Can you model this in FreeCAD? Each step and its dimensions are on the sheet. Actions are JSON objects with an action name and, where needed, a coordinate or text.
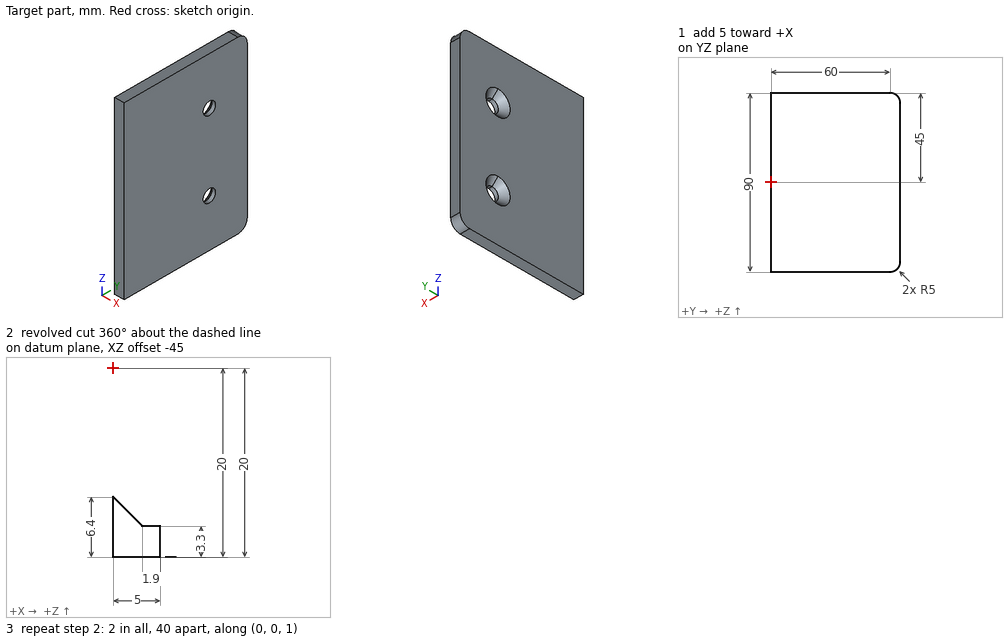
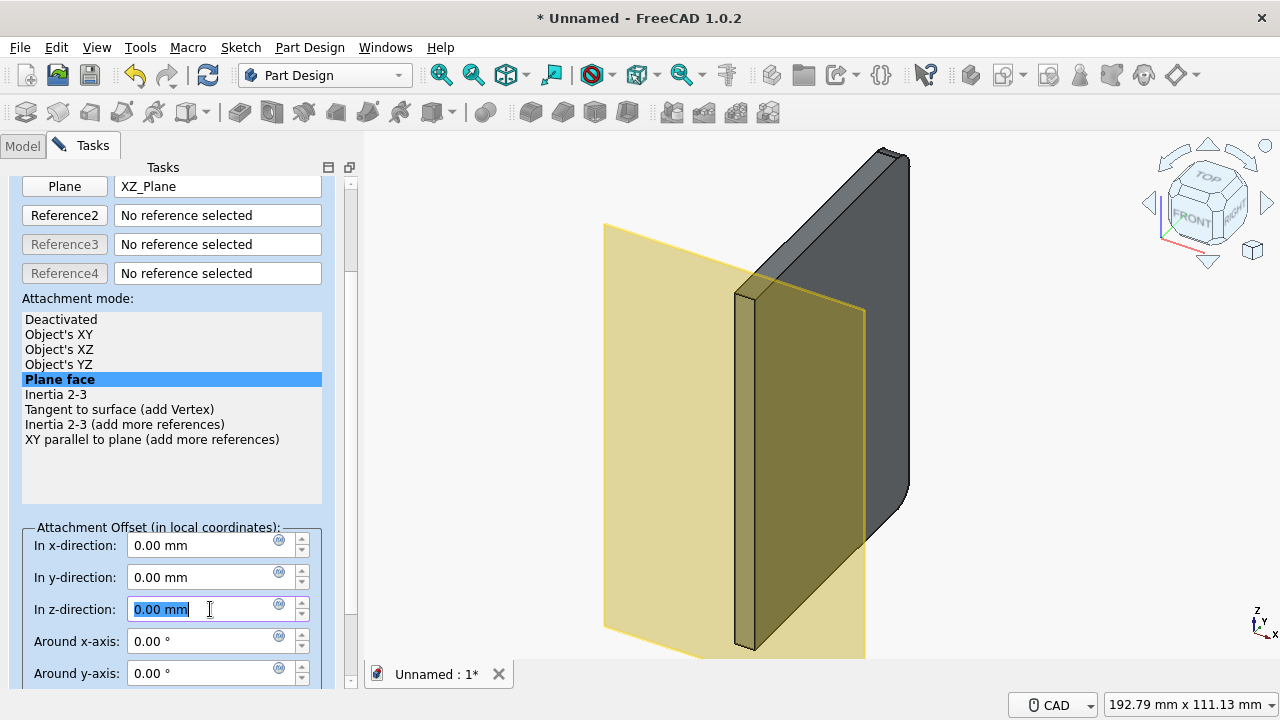
{"action": "type", "text": "-45"}
{"action": "key", "text": "Tab"}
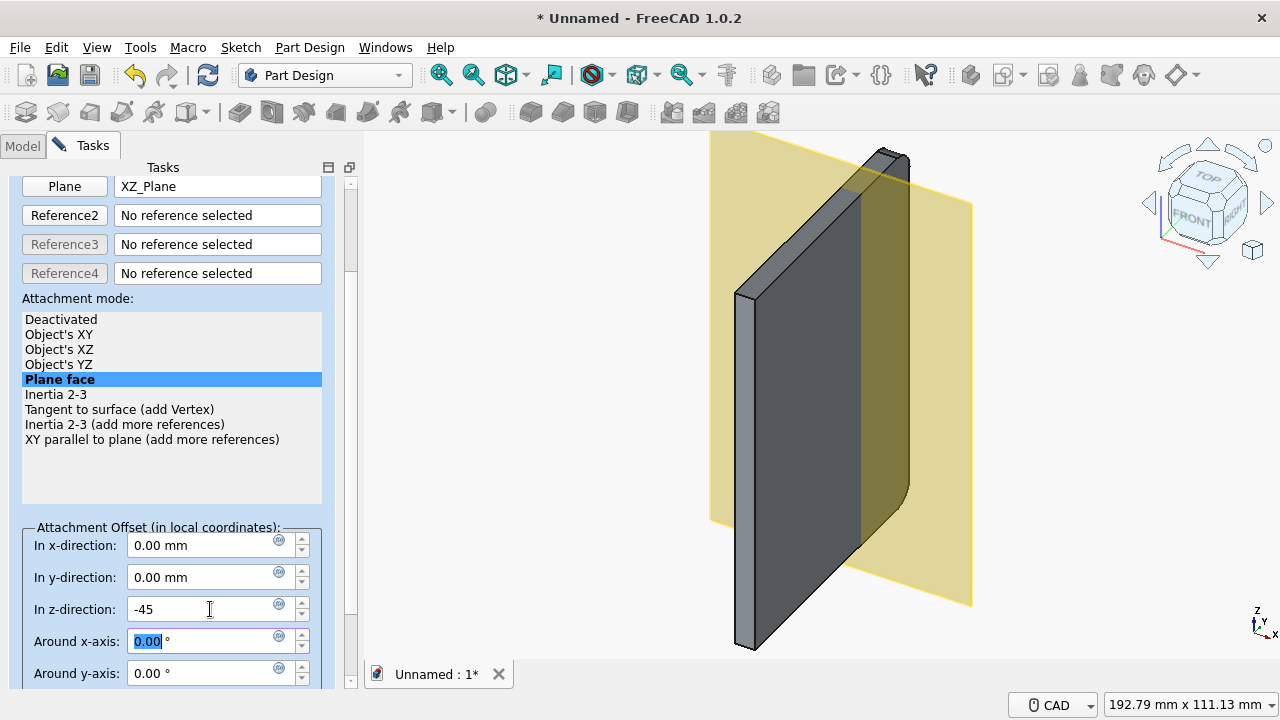
{"action": "scroll", "coordinate": [351, 432], "scroll_direction": "up", "scroll_amount": 3}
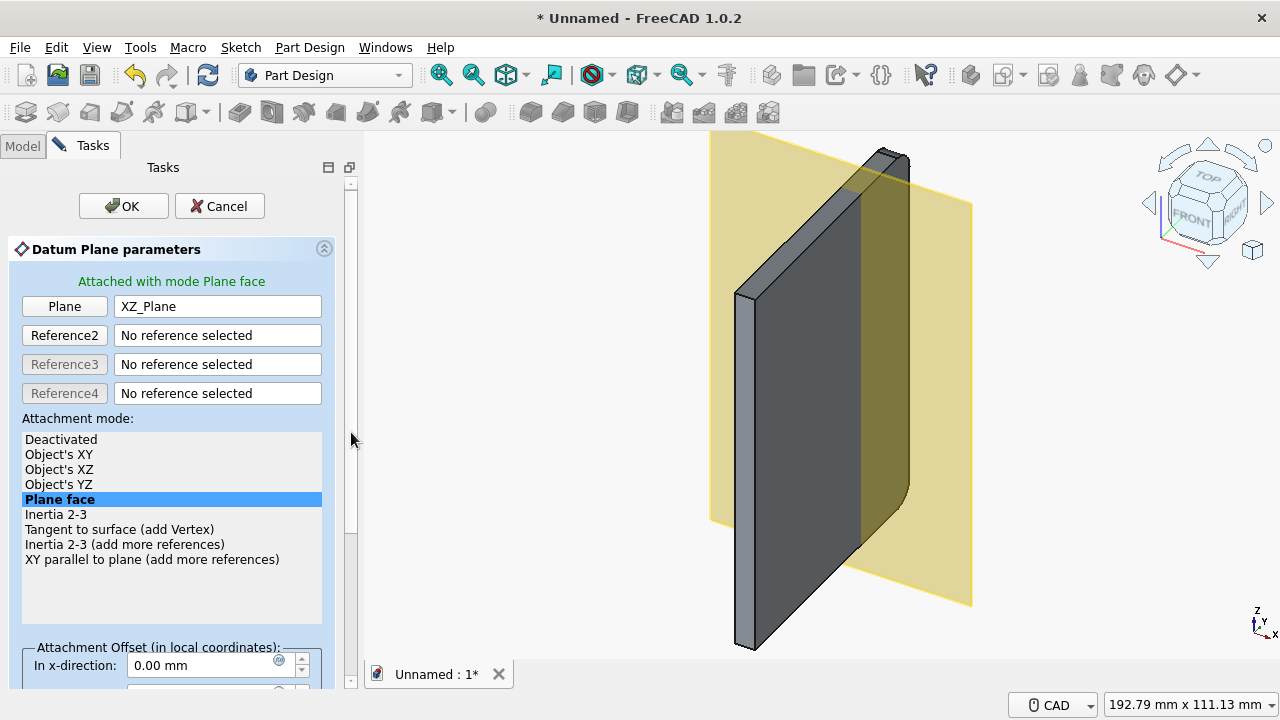
{"action": "left_click", "coordinate": [124, 206]}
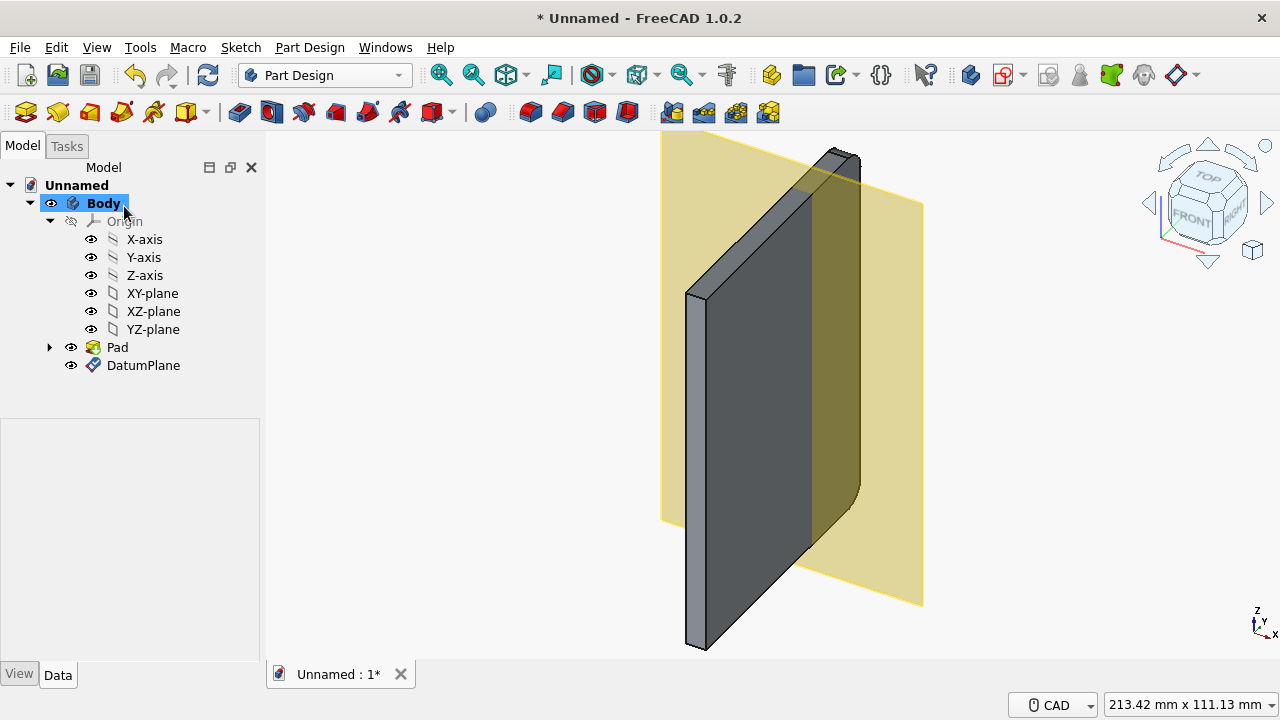
{"action": "left_click", "coordinate": [116, 365]}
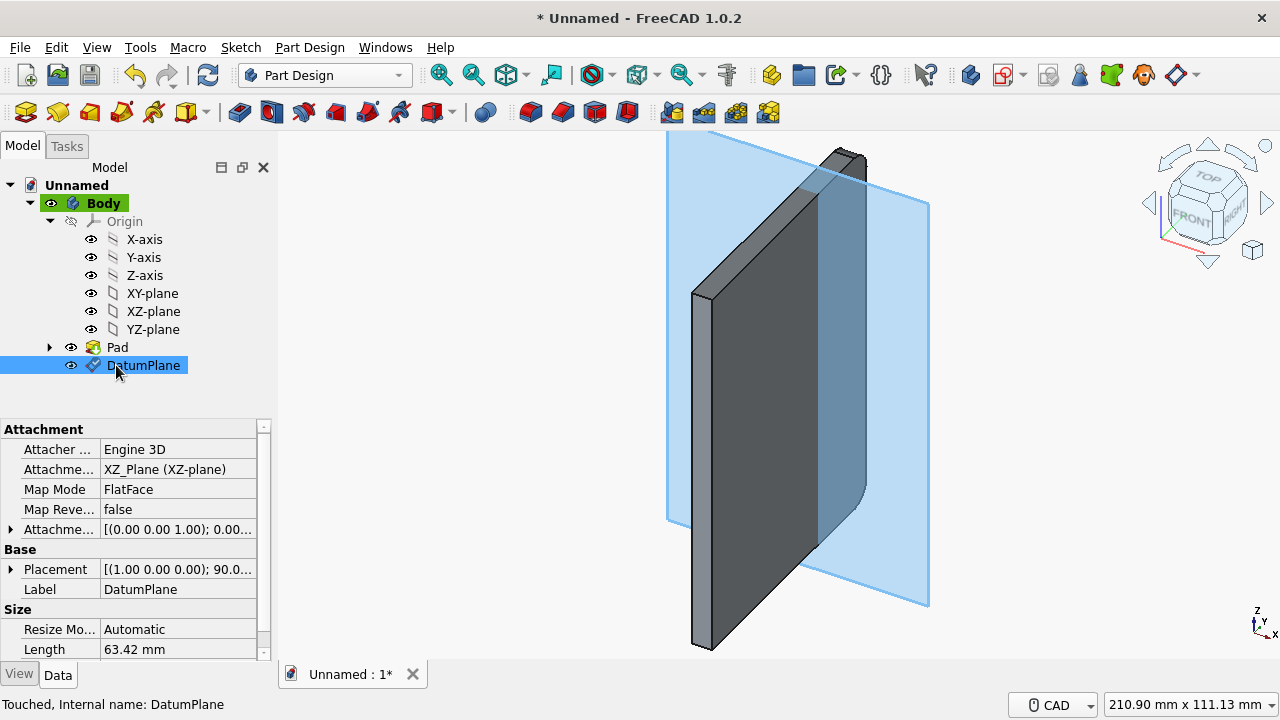
{"action": "left_click", "coordinate": [1004, 76]}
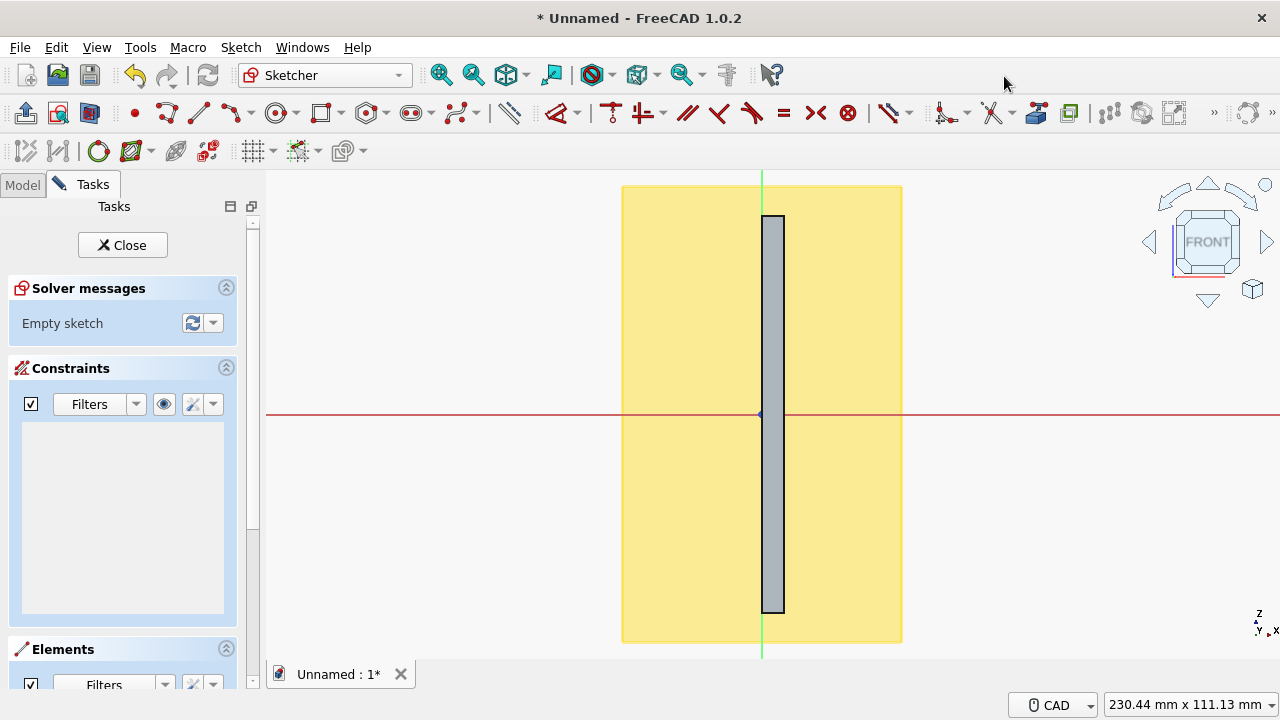
{"action": "left_click", "coordinate": [90, 114]}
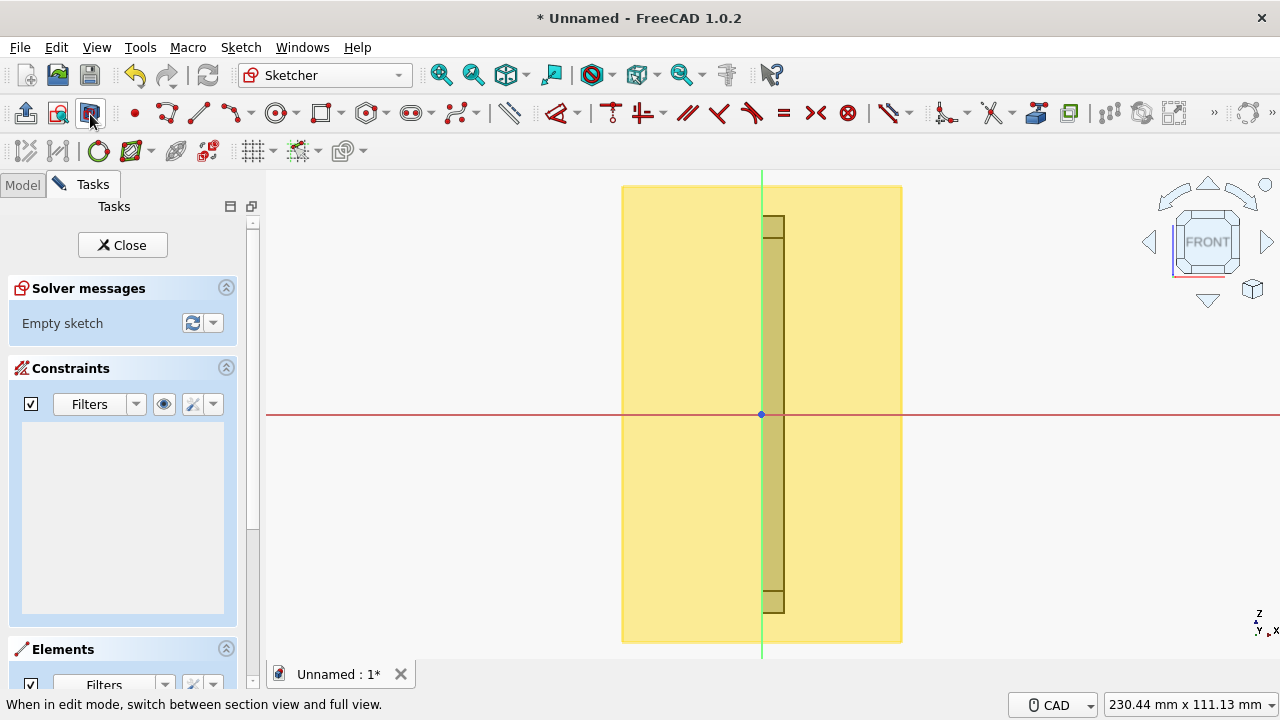
{"action": "scroll", "coordinate": [785, 496], "scroll_direction": "up", "scroll_amount": 12}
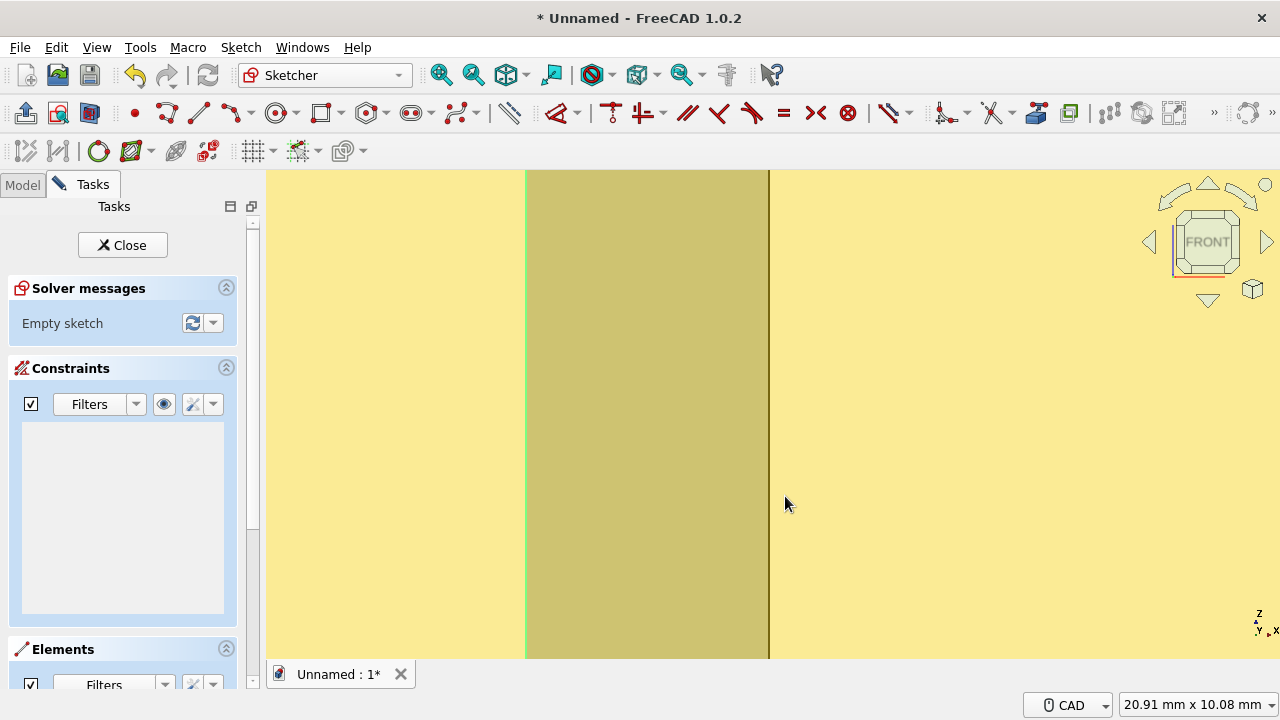
{"action": "left_click", "coordinate": [168, 114]}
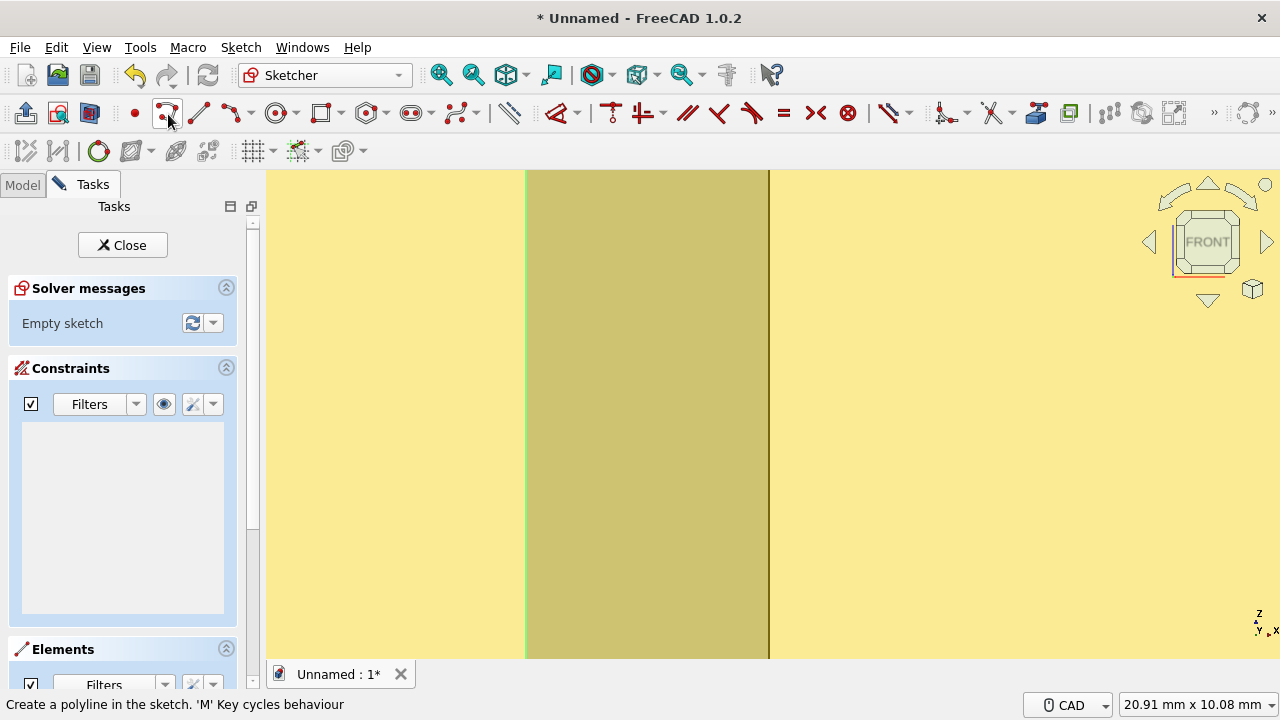
{"action": "left_click", "coordinate": [526, 251]}
{"action": "left_click", "coordinate": [677, 401]}
{"action": "left_click", "coordinate": [769, 401]}
{"action": "left_click", "coordinate": [769, 561]}
{"action": "left_click", "coordinate": [535, 561]}
{"action": "left_click", "coordinate": [526, 252]}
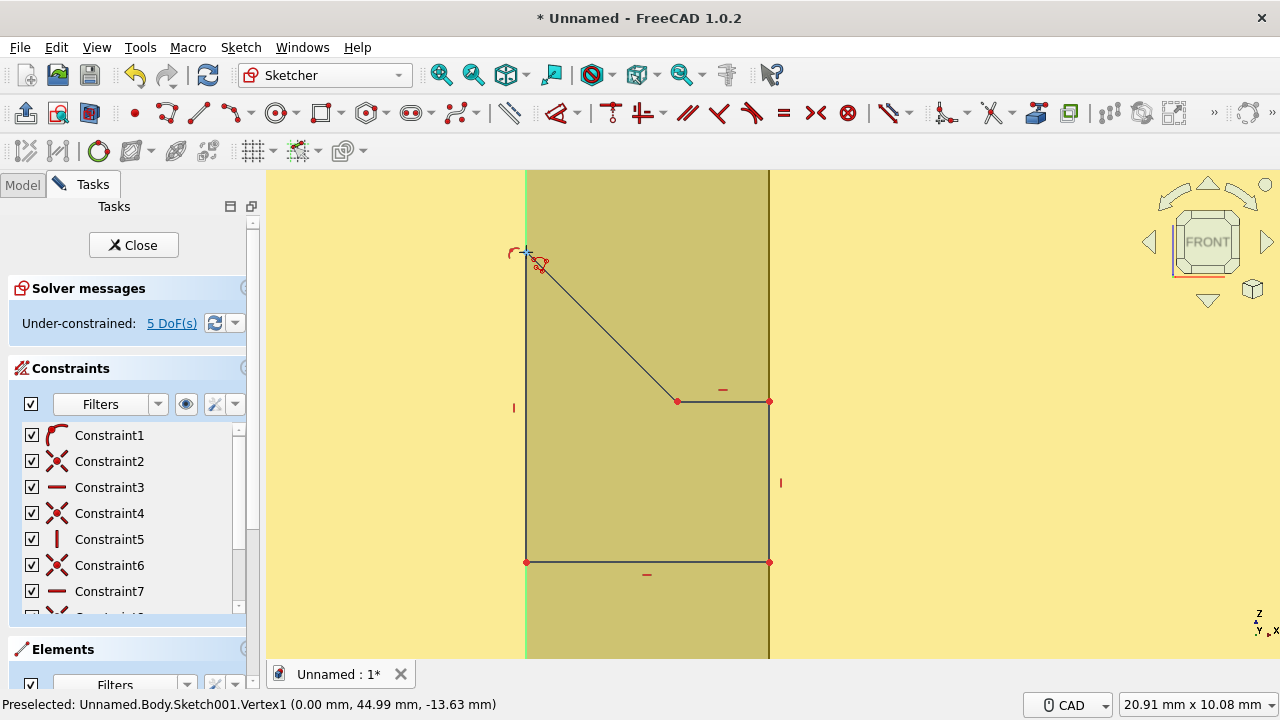
{"action": "left_click", "coordinate": [200, 114]}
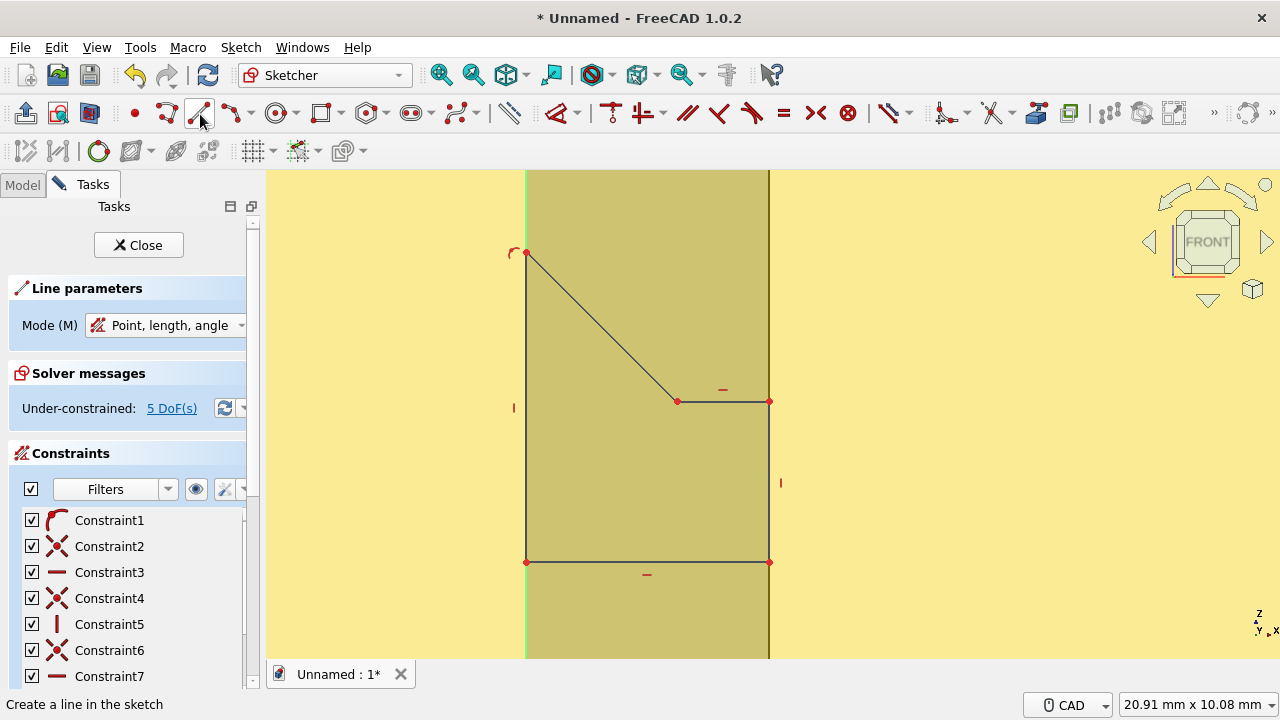
{"action": "left_click", "coordinate": [793, 561]}
{"action": "left_click", "coordinate": [866, 561]}
{"action": "key", "text": "Escape"}